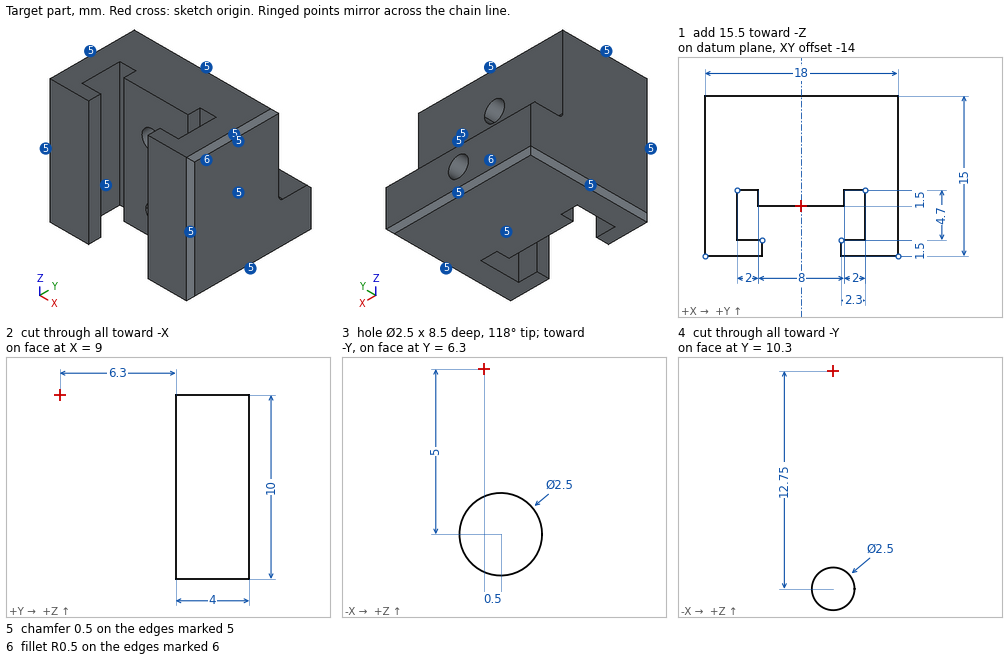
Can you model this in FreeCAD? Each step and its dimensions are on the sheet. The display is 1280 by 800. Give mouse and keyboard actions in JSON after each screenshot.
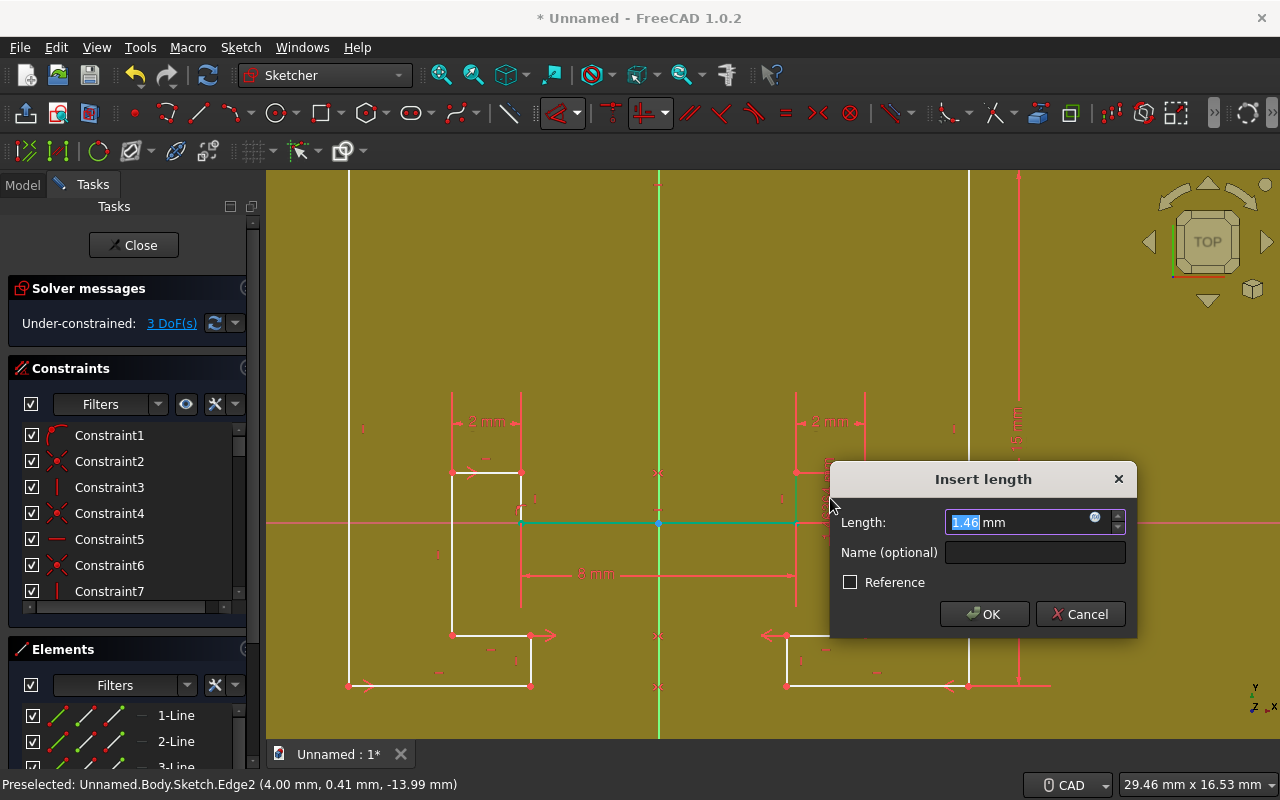
{"action": "type", "text": "1.5"}
{"action": "key", "text": "Return"}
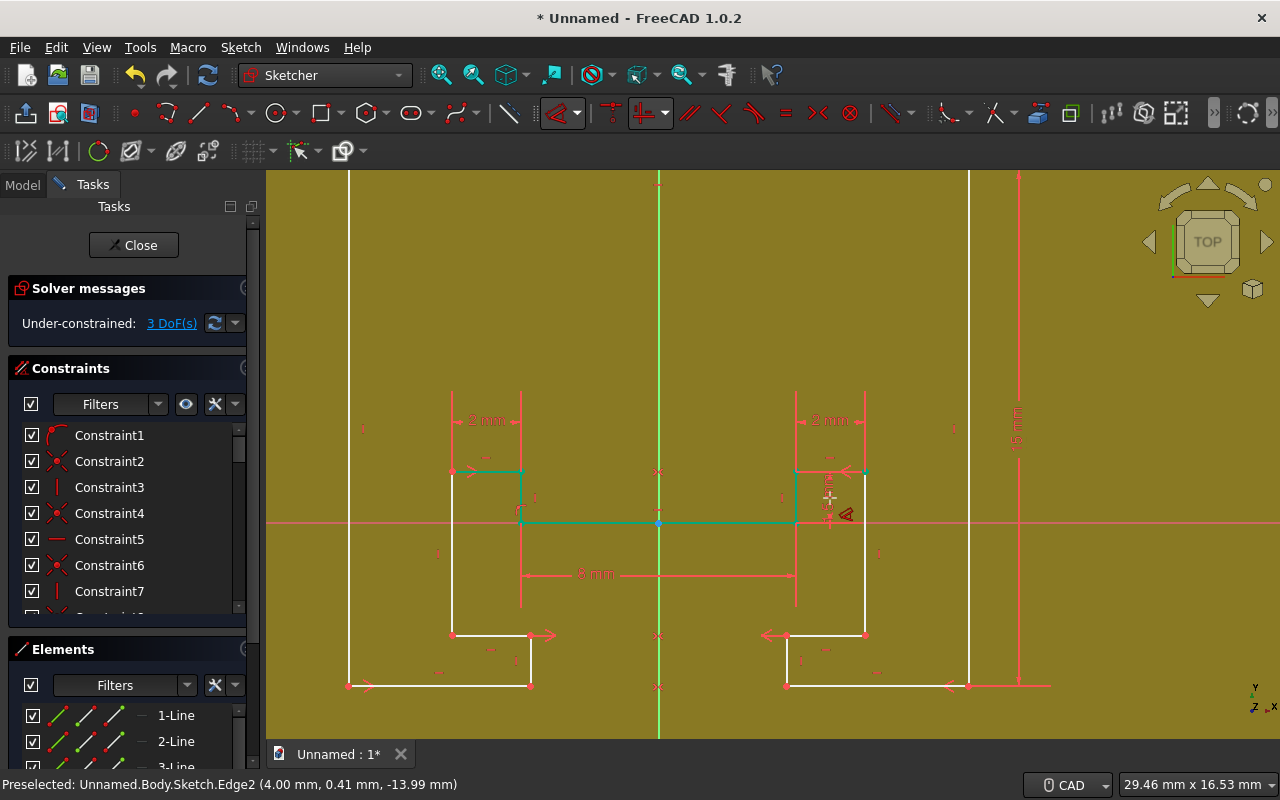
{"action": "left_click", "coordinate": [865, 521]}
{"action": "left_click", "coordinate": [899, 554]}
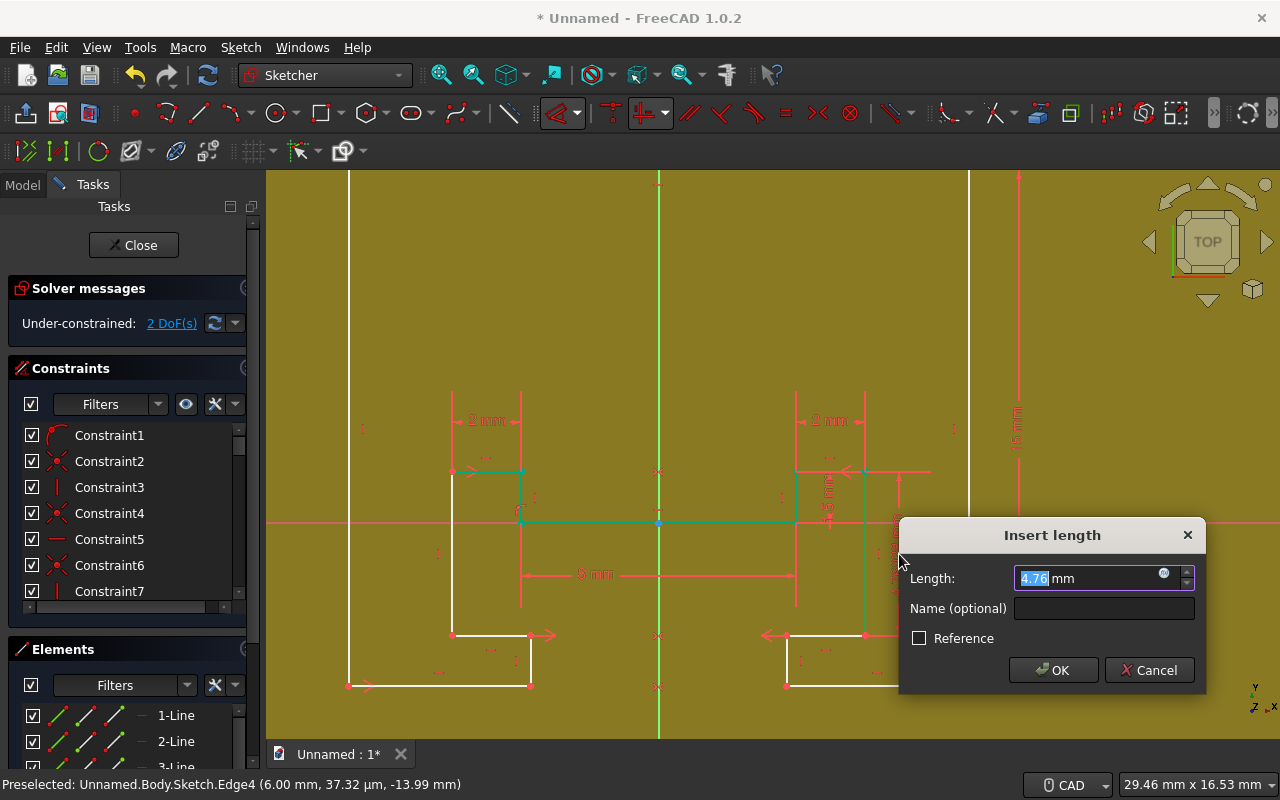
{"action": "type", "text": "4.7"}
{"action": "key", "text": "Return"}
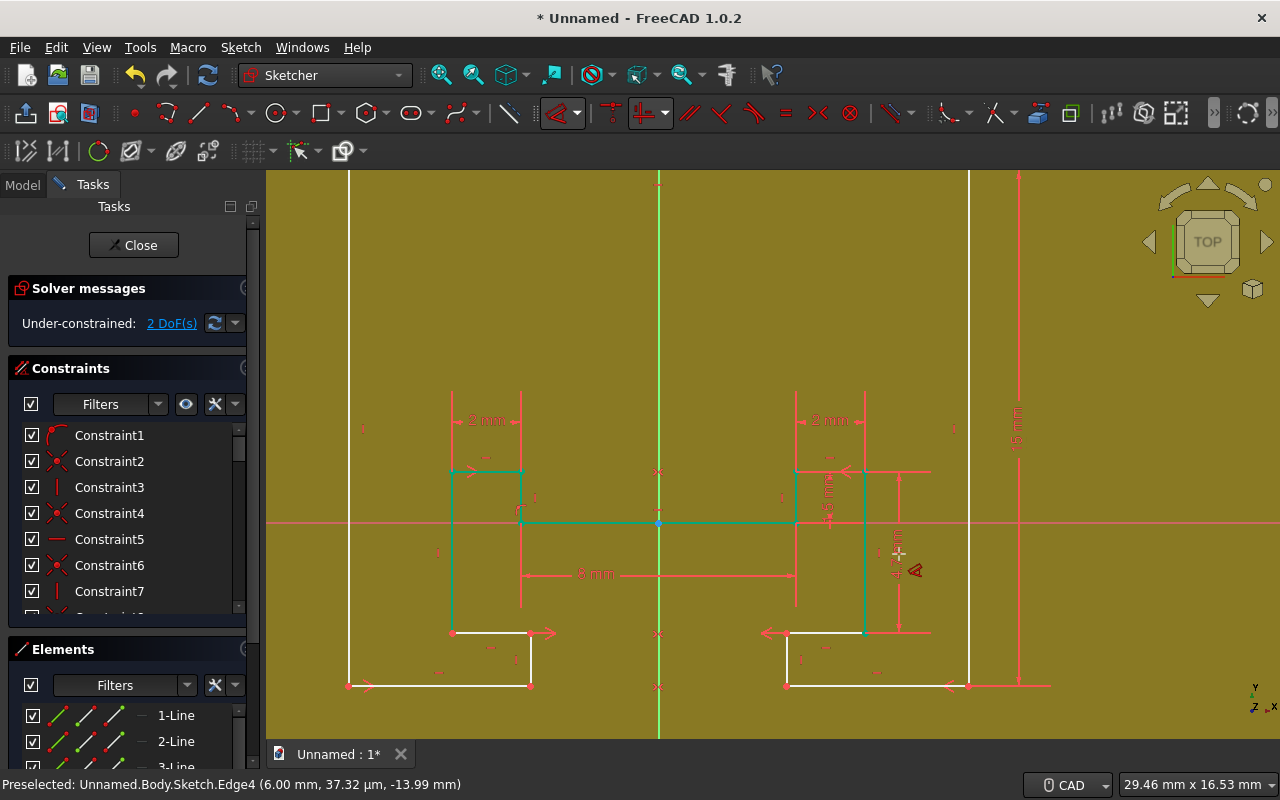
{"action": "left_click", "coordinate": [842, 633]}
{"action": "left_click", "coordinate": [826, 667]}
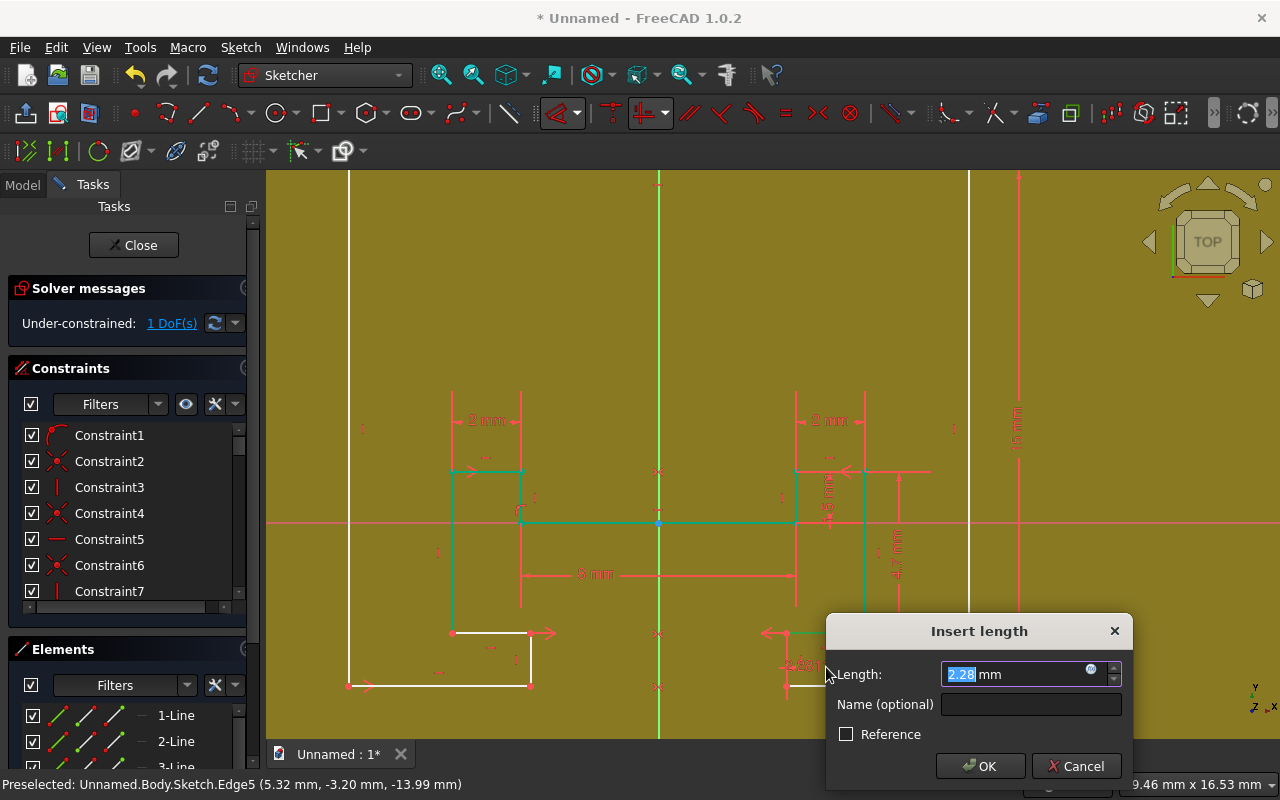
{"action": "type", "text": "2.3"}
{"action": "key", "text": "Return"}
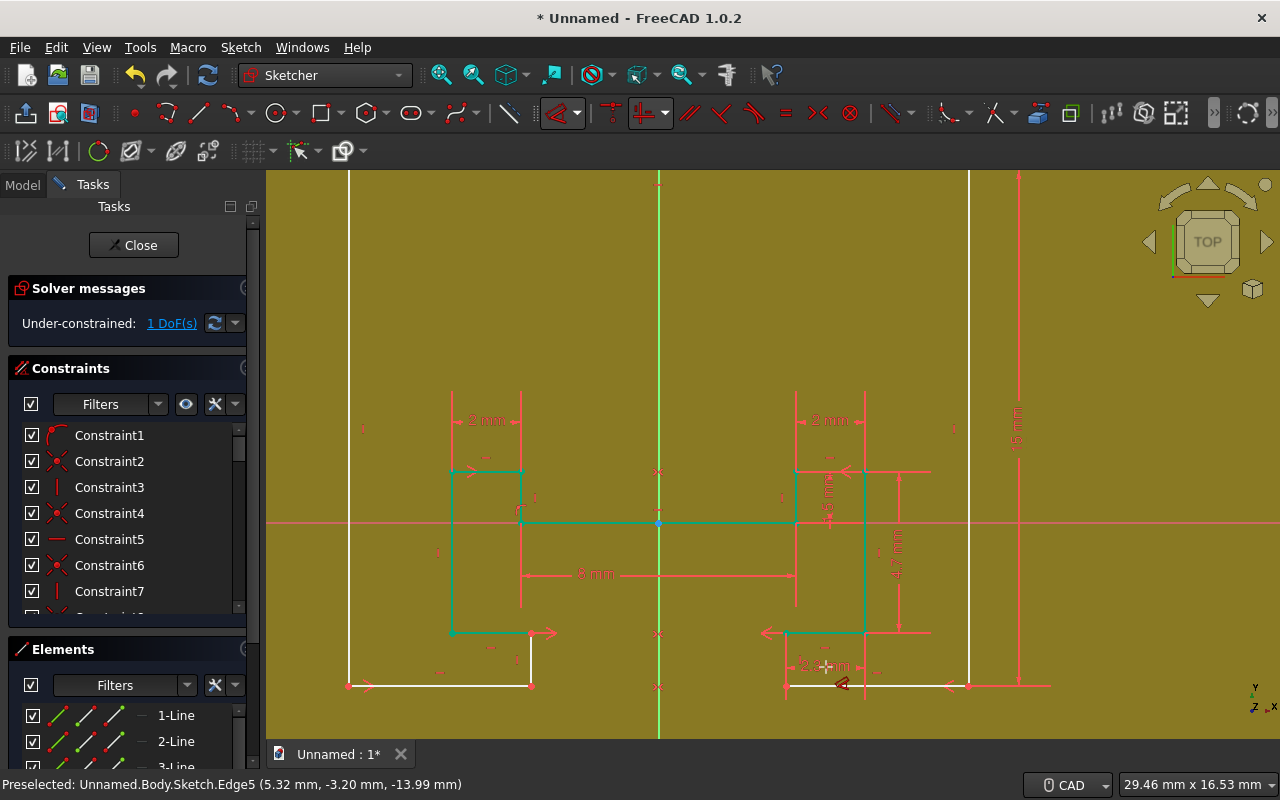
{"action": "left_click", "coordinate": [786, 649]}
{"action": "left_click", "coordinate": [752, 660]}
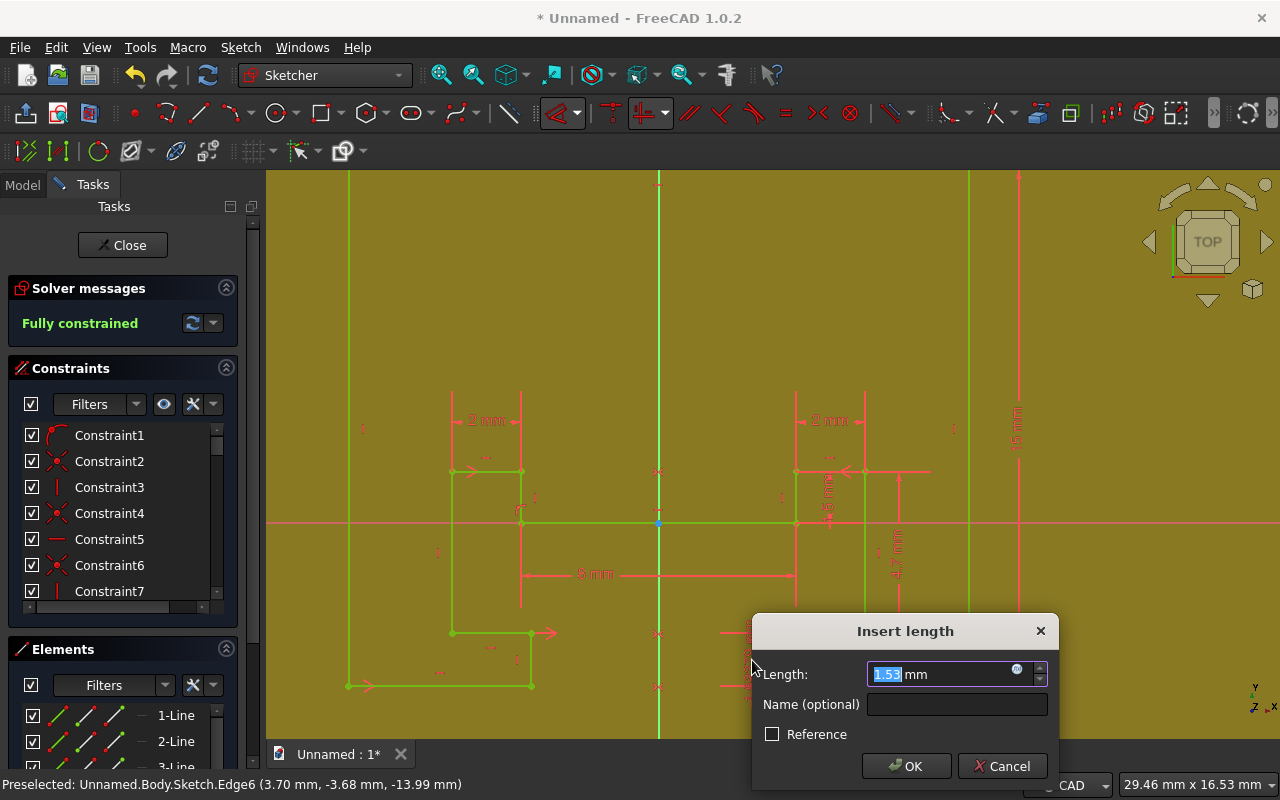
{"action": "type", "text": "1.5"}
{"action": "key", "text": "Return"}
{"action": "key", "text": "Escape"}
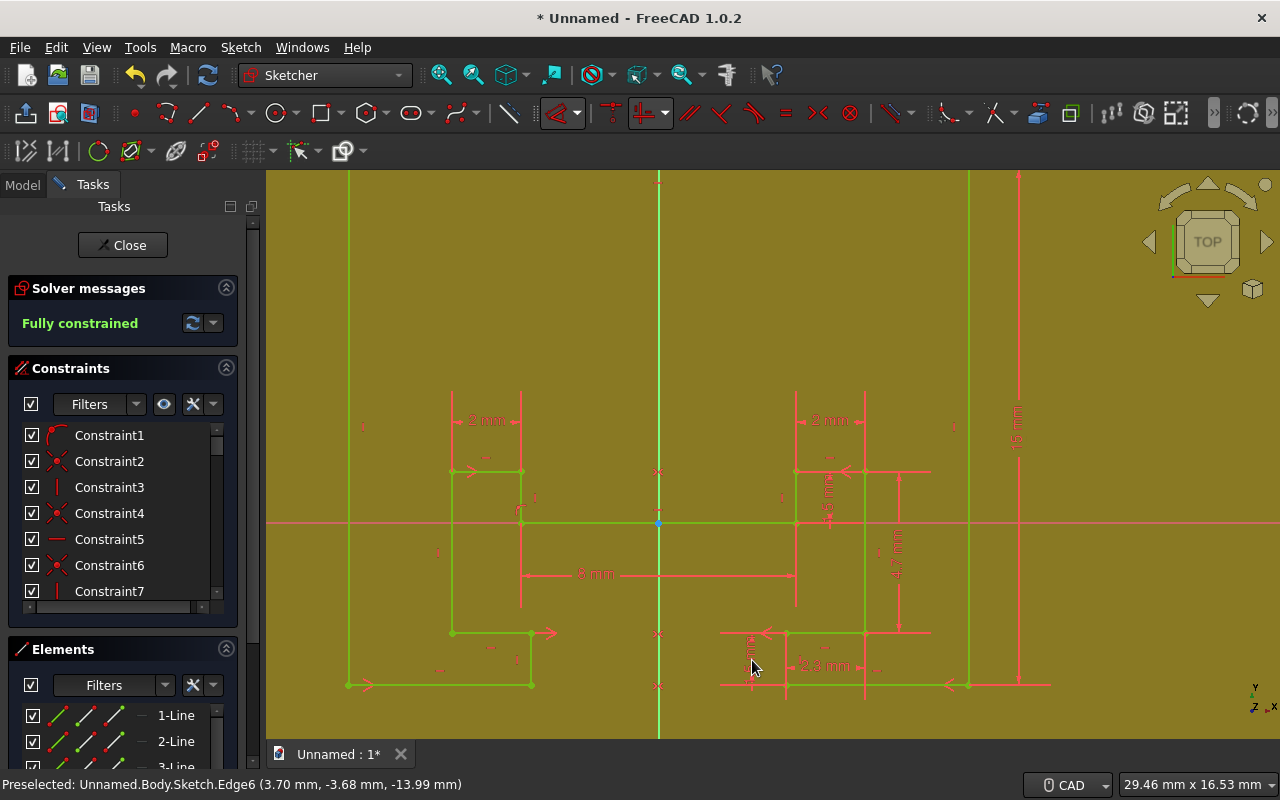
{"action": "left_click", "coordinate": [123, 245]}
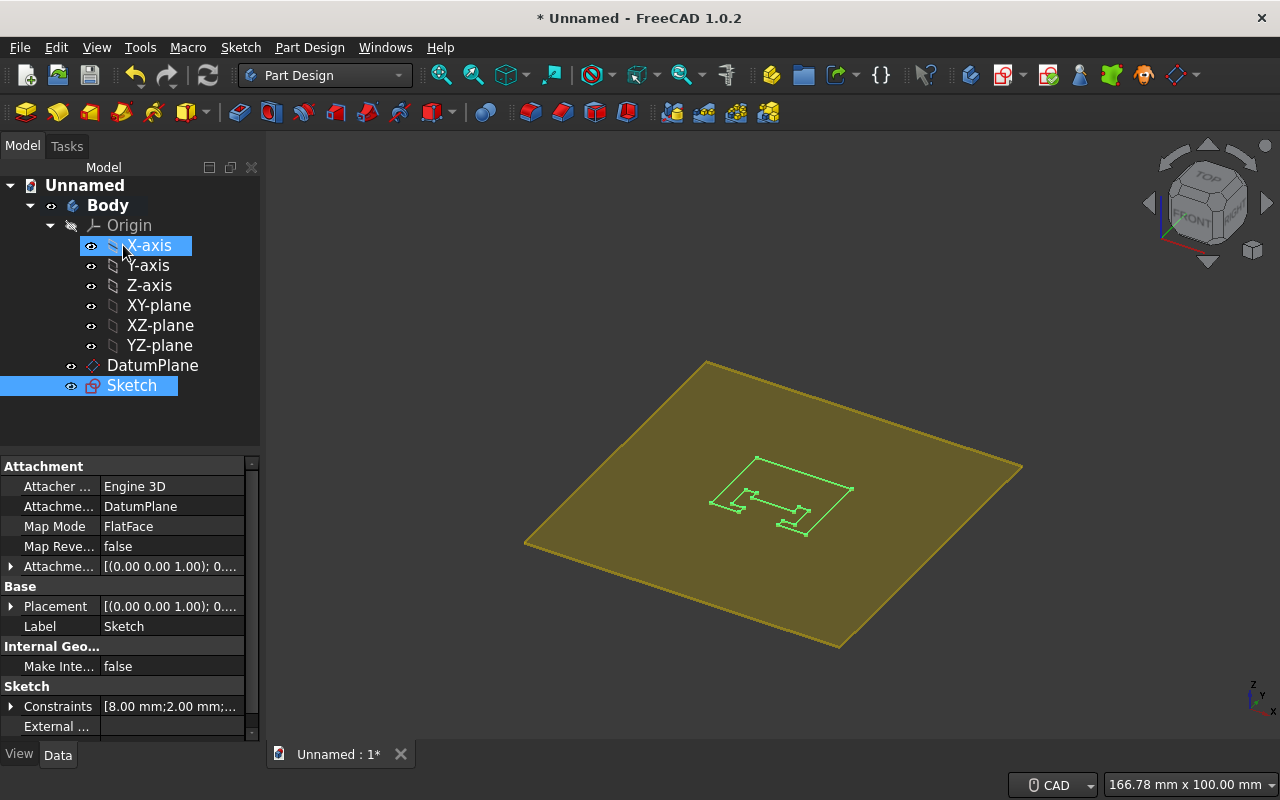
{"action": "left_click", "coordinate": [26, 112]}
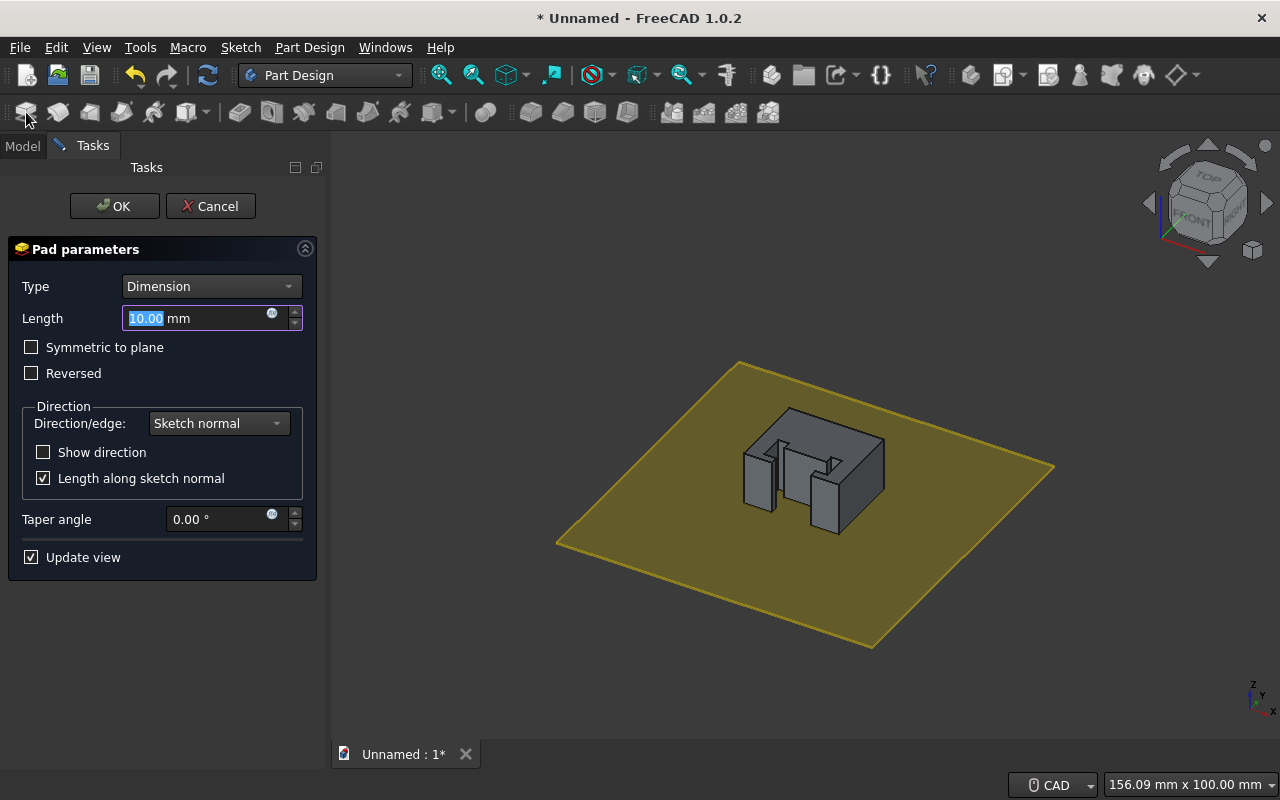
{"action": "type", "text": "15.5"}
{"action": "key", "text": "Tab"}